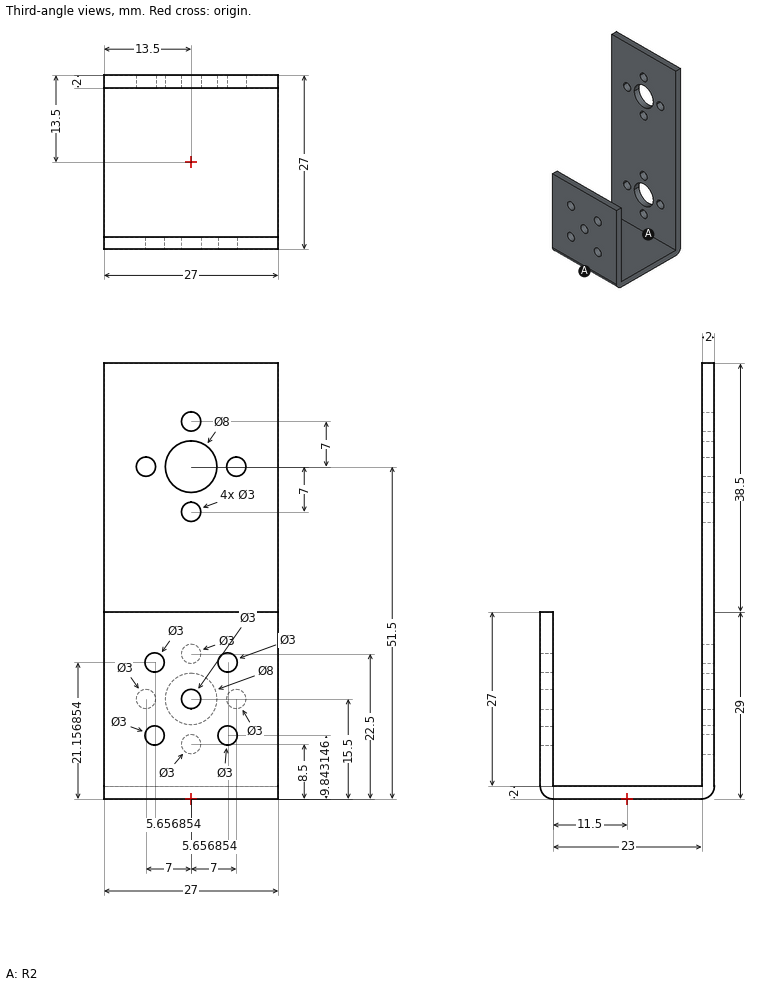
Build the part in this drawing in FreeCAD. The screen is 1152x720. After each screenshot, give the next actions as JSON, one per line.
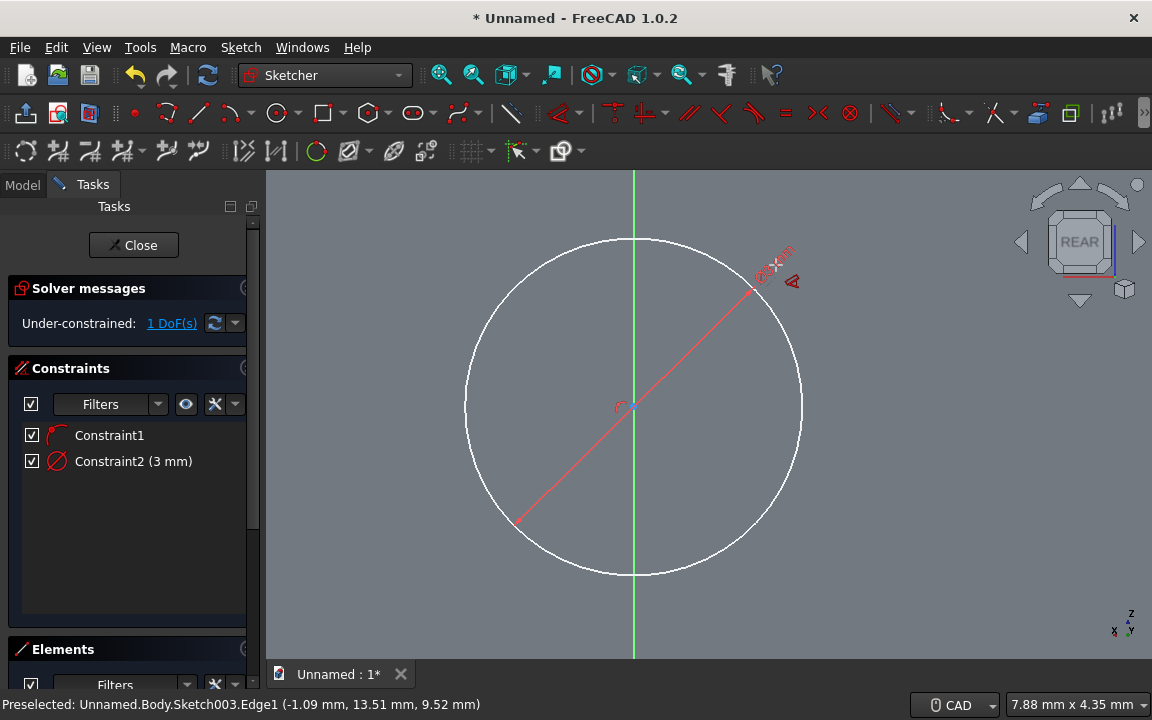
{"action": "left_click", "coordinate": [634, 407]}
{"action": "left_click", "coordinate": [668, 519]}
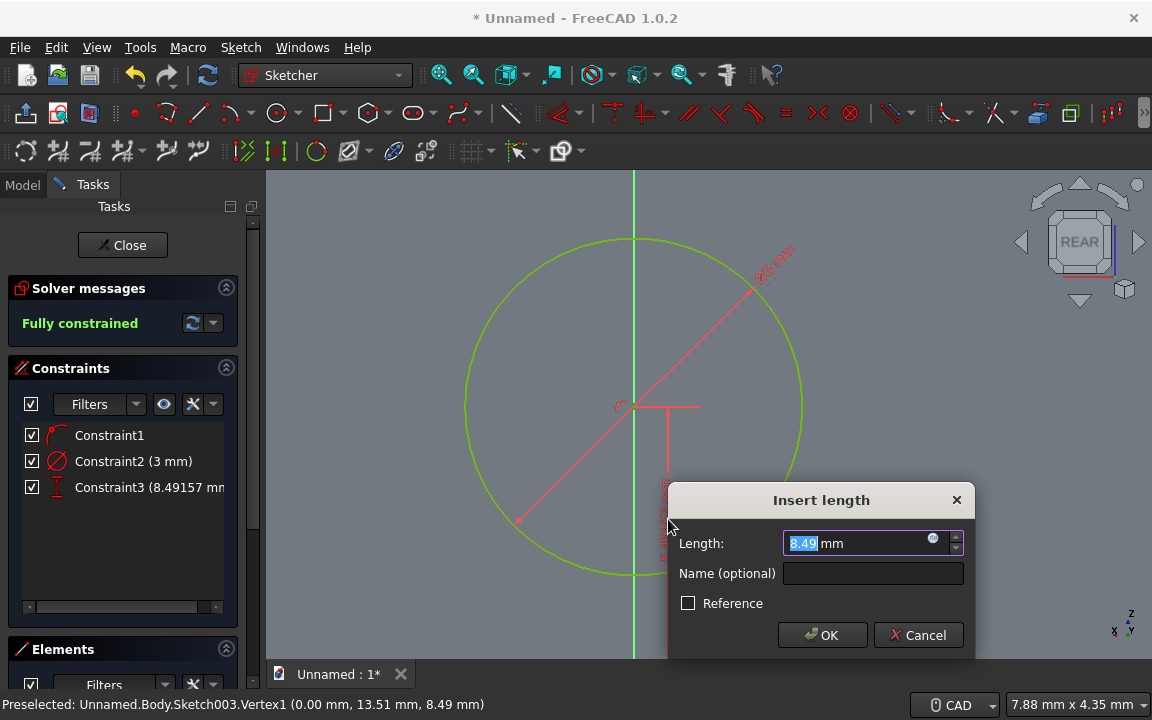
{"action": "type", "text": "8.5"}
{"action": "key", "text": "Return"}
{"action": "key", "text": "Escape"}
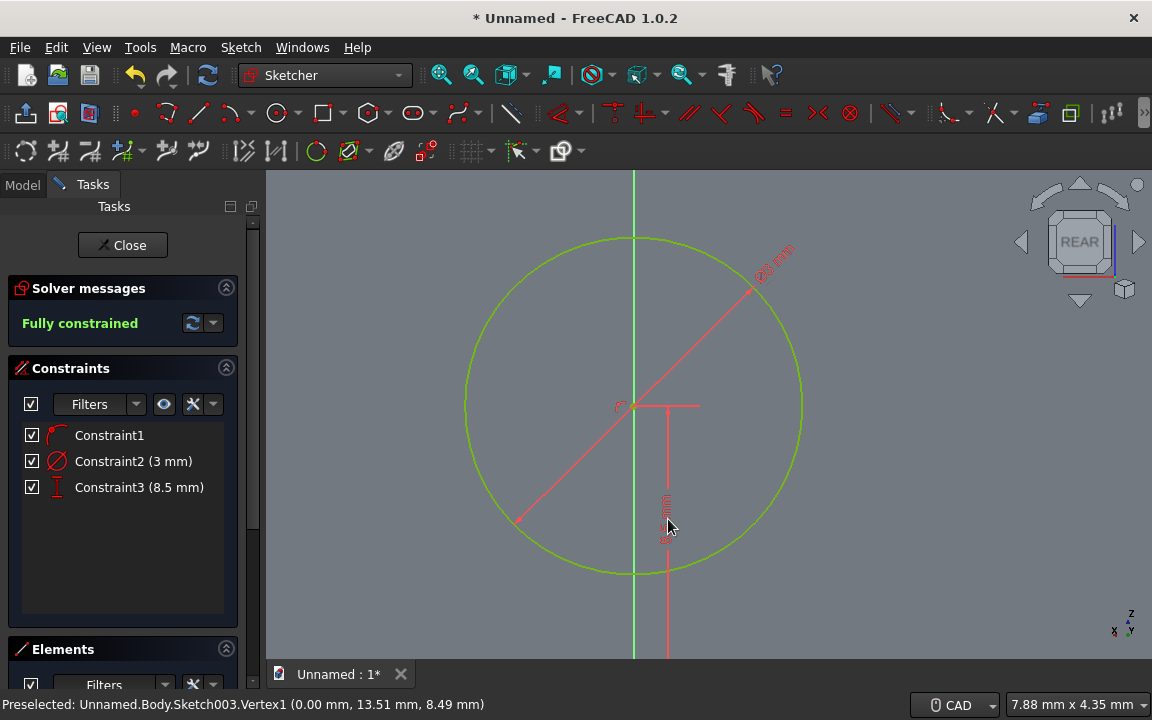
{"action": "left_click", "coordinate": [123, 245]}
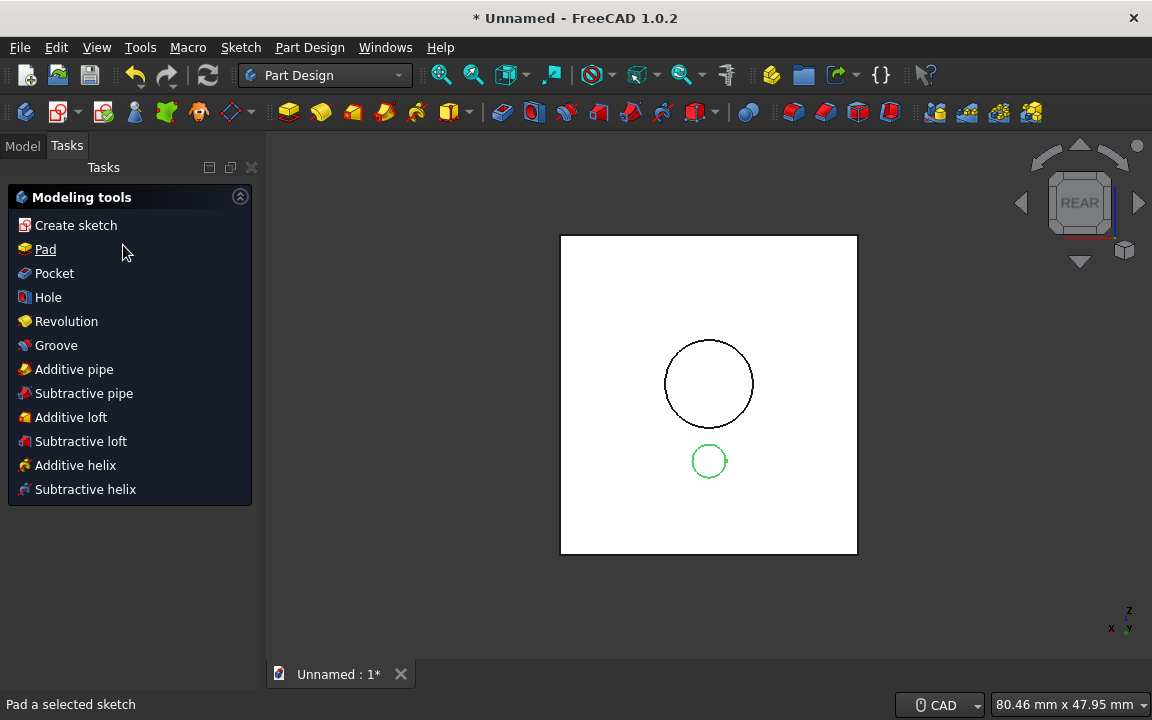
{"action": "left_click", "coordinate": [504, 112]}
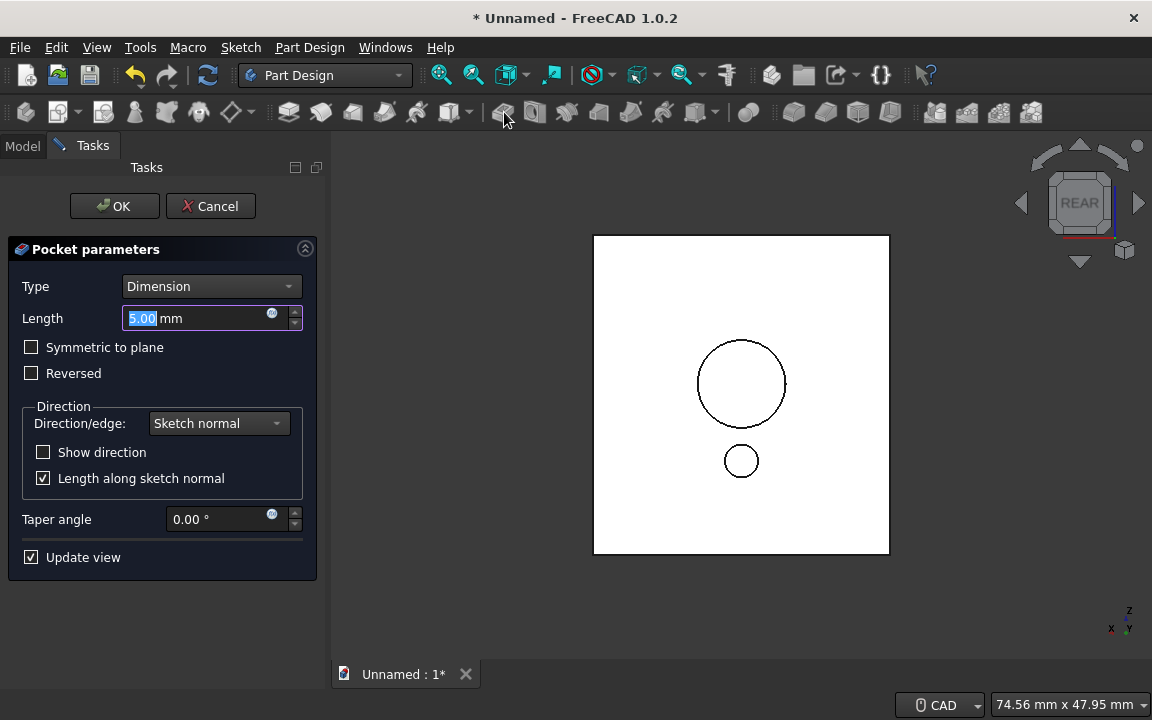
{"action": "left_click", "coordinate": [212, 286]}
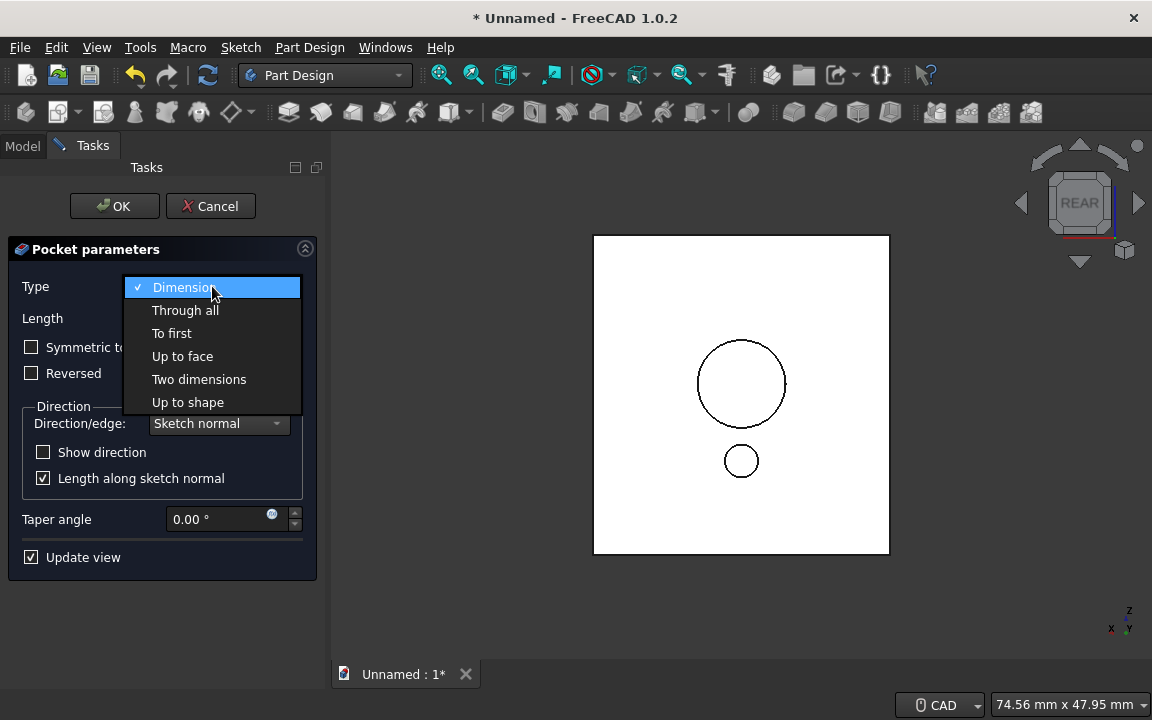
{"action": "left_click", "coordinate": [212, 334]}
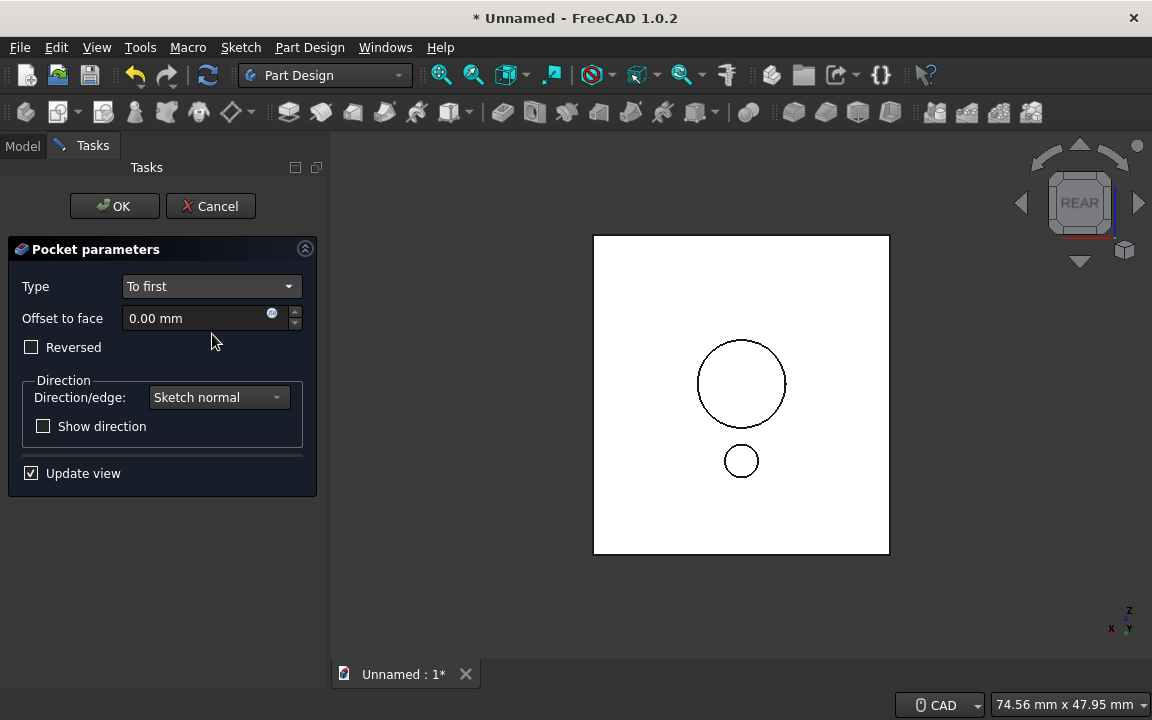
{"action": "left_click", "coordinate": [115, 206]}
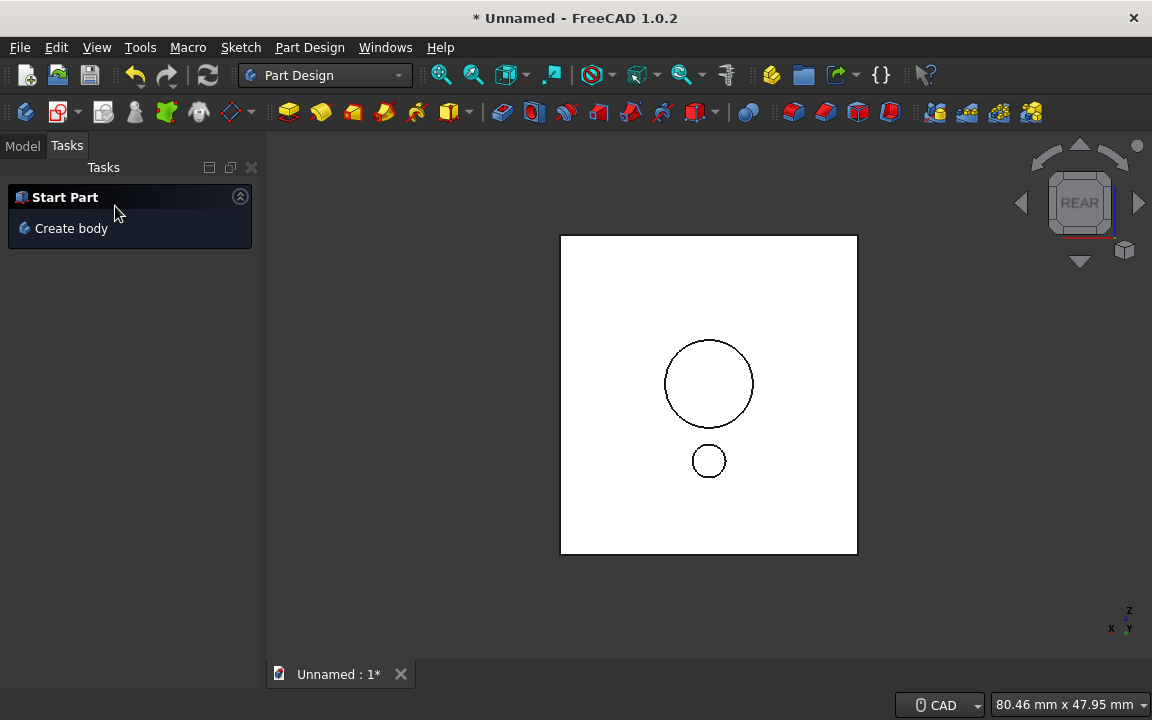
{"action": "left_click", "coordinate": [624, 303]}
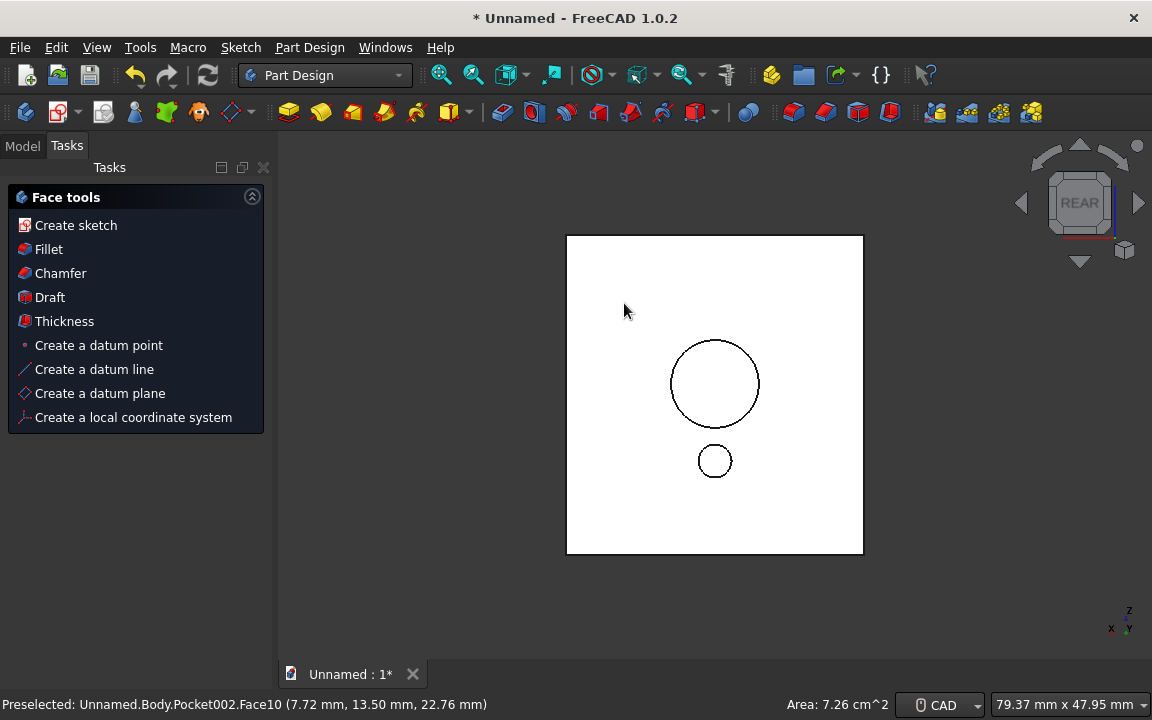
{"action": "left_click", "coordinate": [58, 112]}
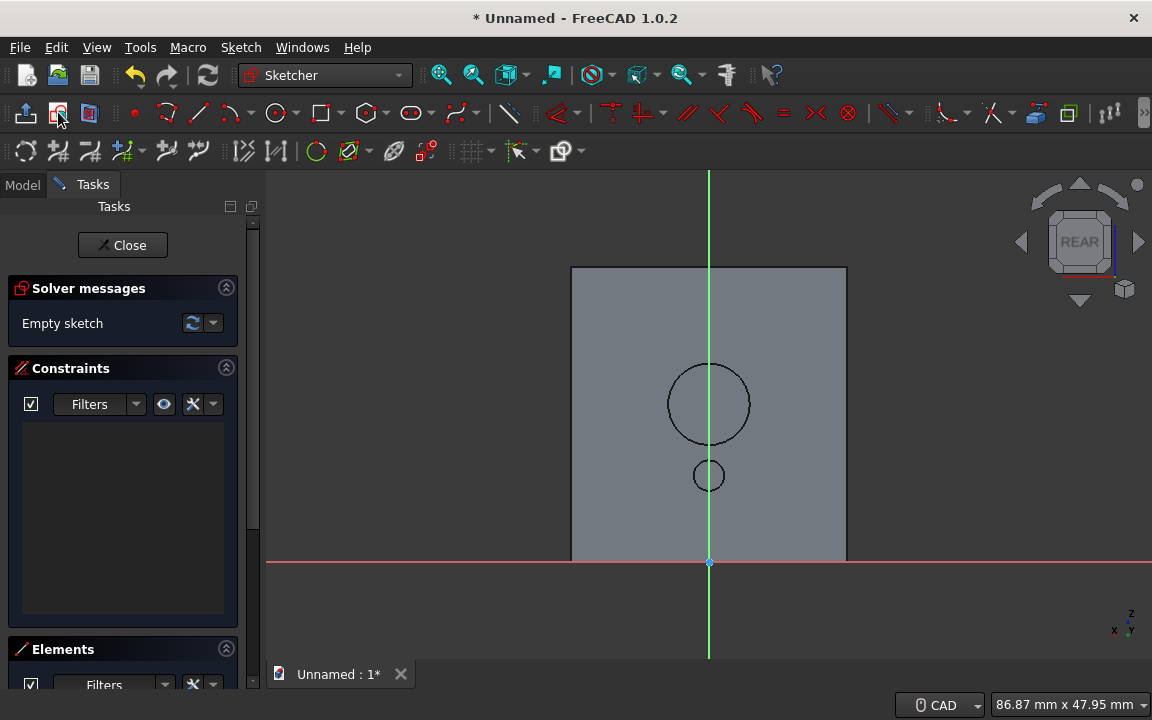
{"action": "scroll", "coordinate": [637, 403], "scroll_direction": "up", "scroll_amount": 12}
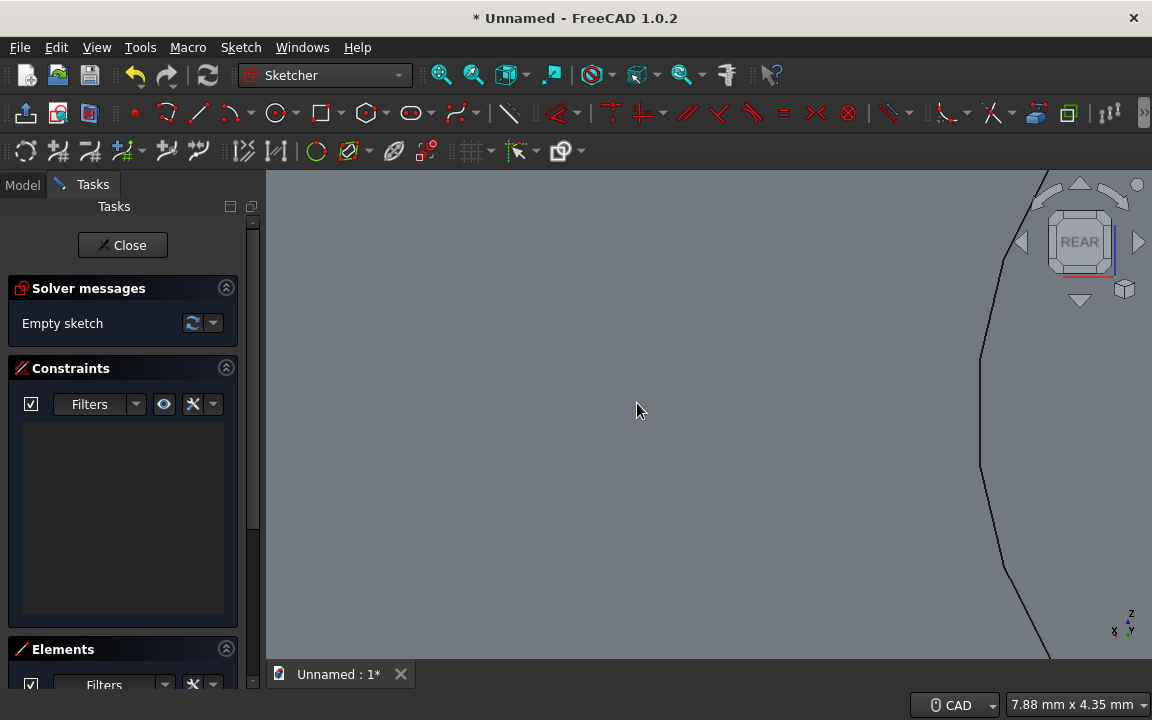
{"action": "key", "text": "g c"}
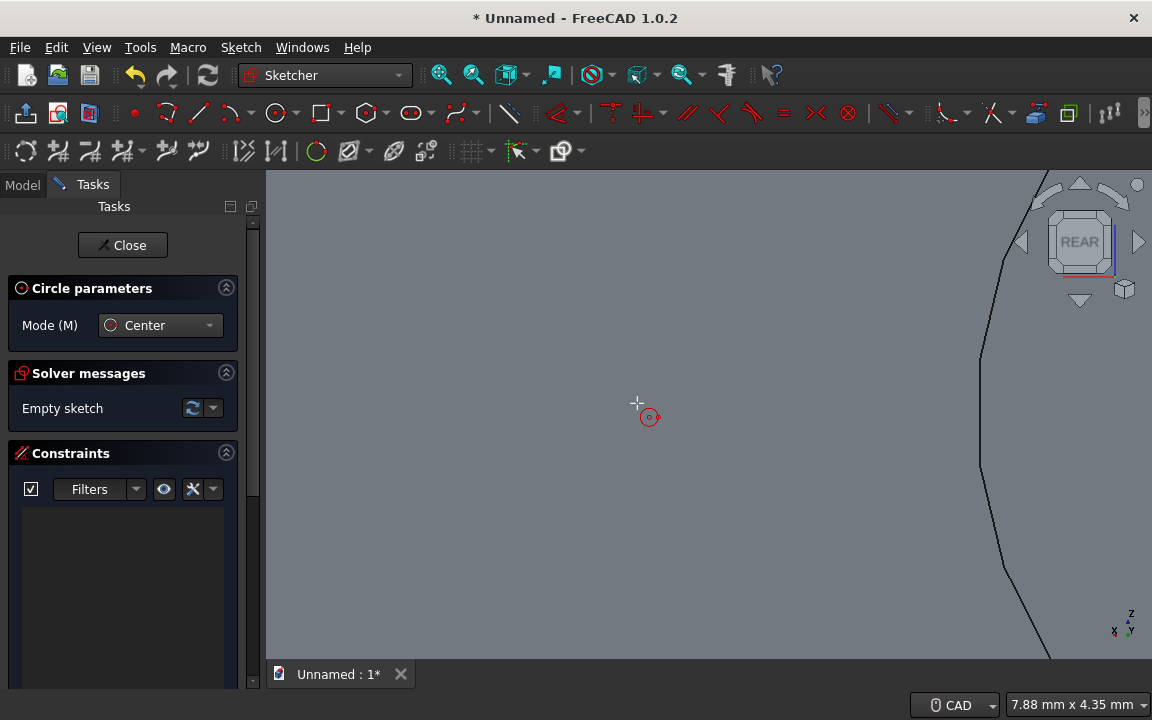
{"action": "left_click", "coordinate": [640, 413]}
{"action": "left_click", "coordinate": [759, 293]}
{"action": "key", "text": "Escape"}